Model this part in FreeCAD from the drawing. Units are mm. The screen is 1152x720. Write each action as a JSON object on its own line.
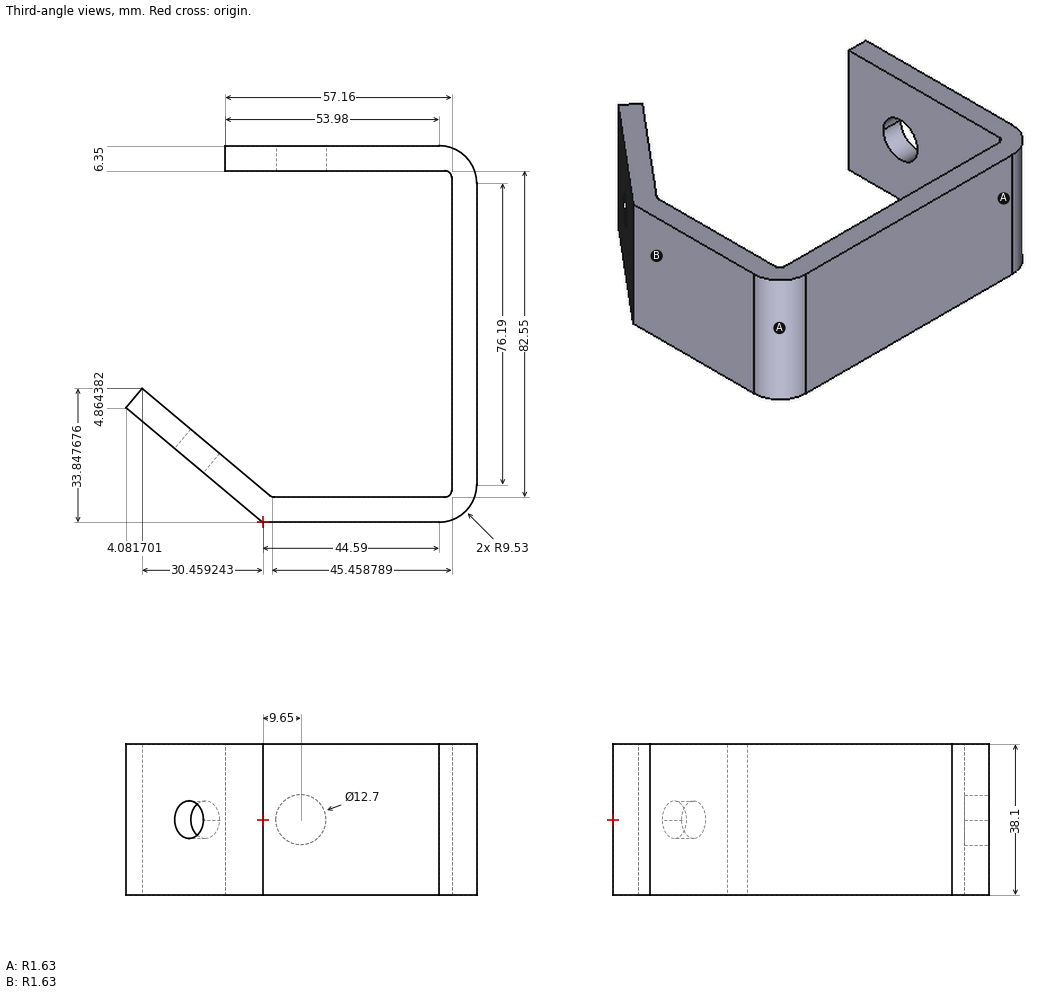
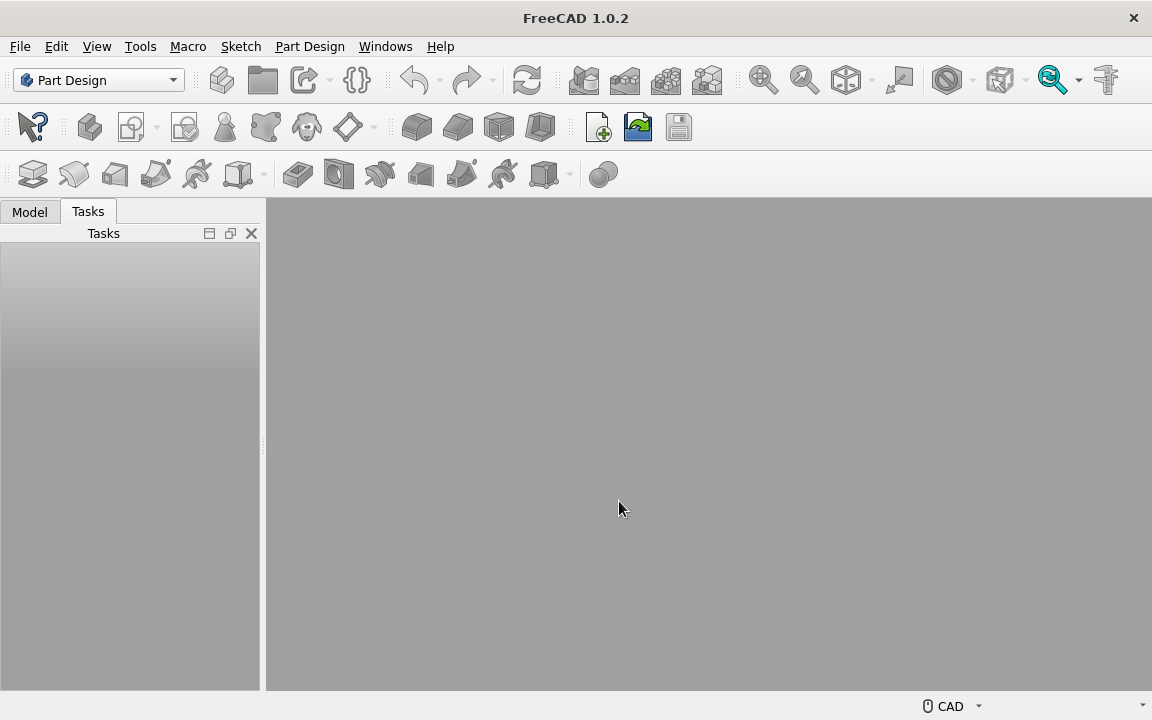
{"action": "key", "text": "ctrl+n"}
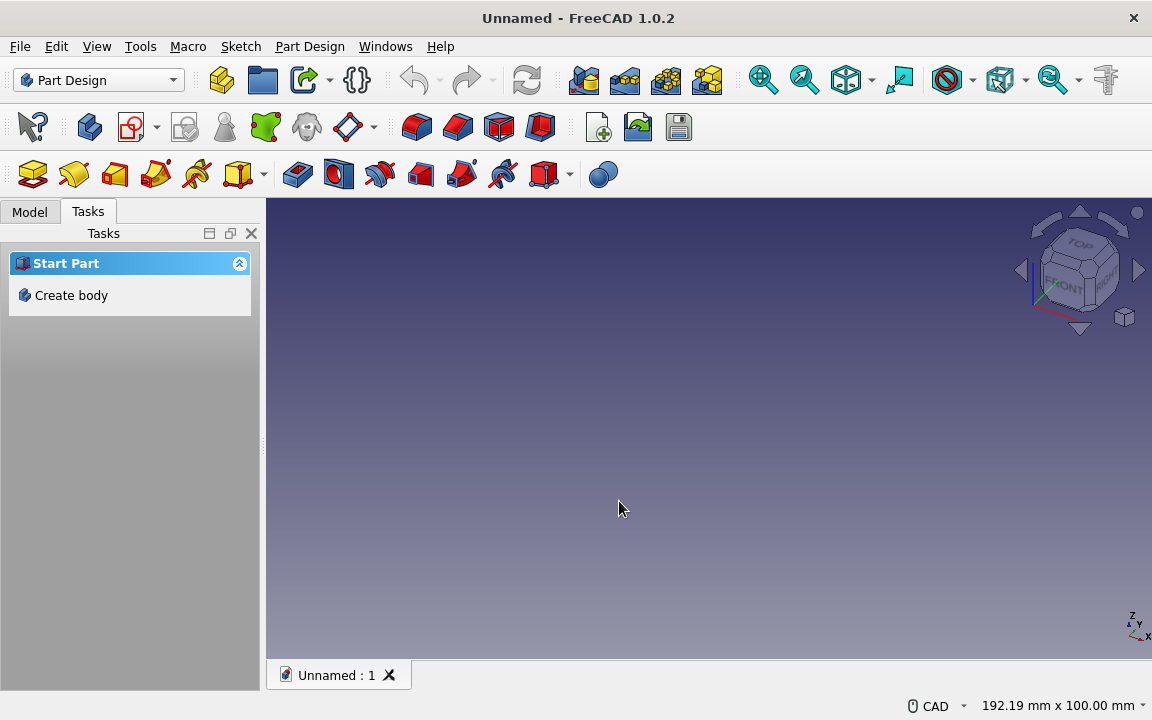
{"action": "left_click", "coordinate": [130, 128]}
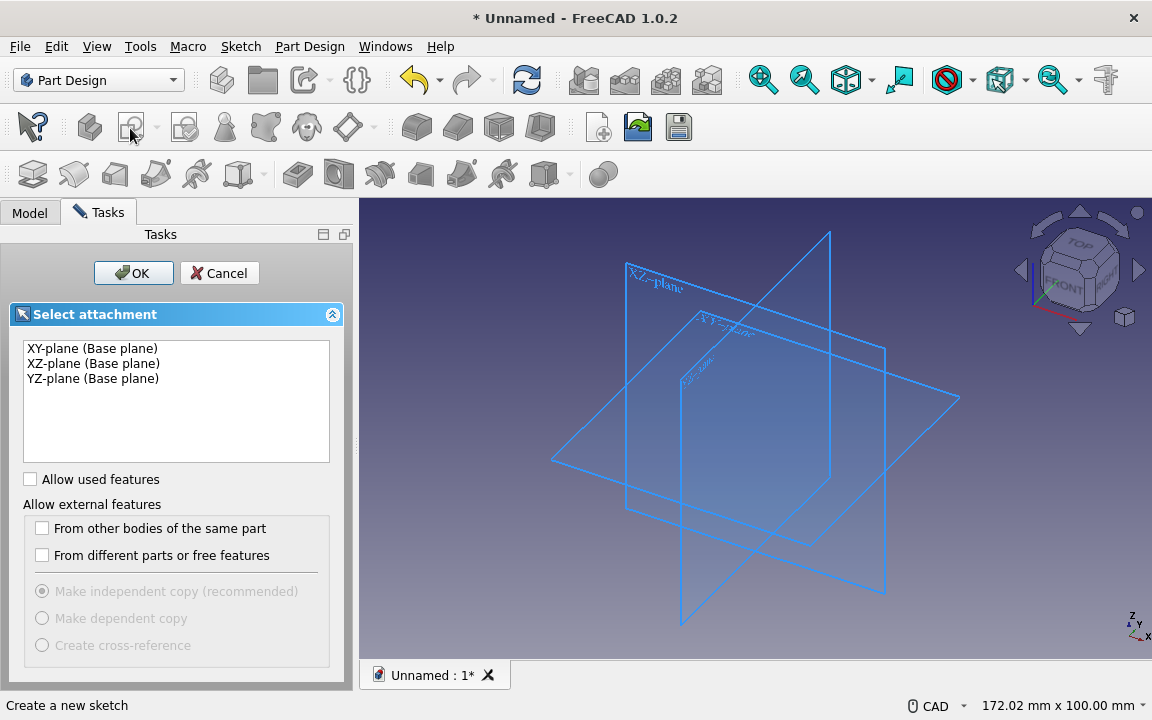
{"action": "left_click", "coordinate": [84, 348]}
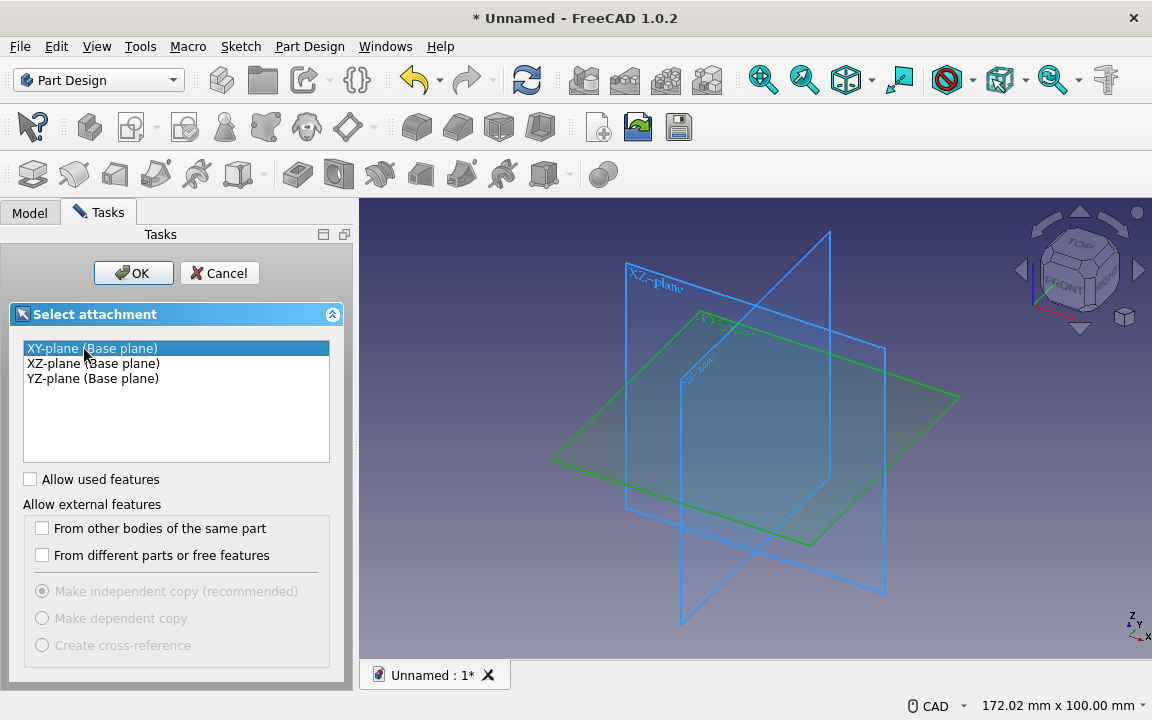
{"action": "left_click", "coordinate": [134, 273]}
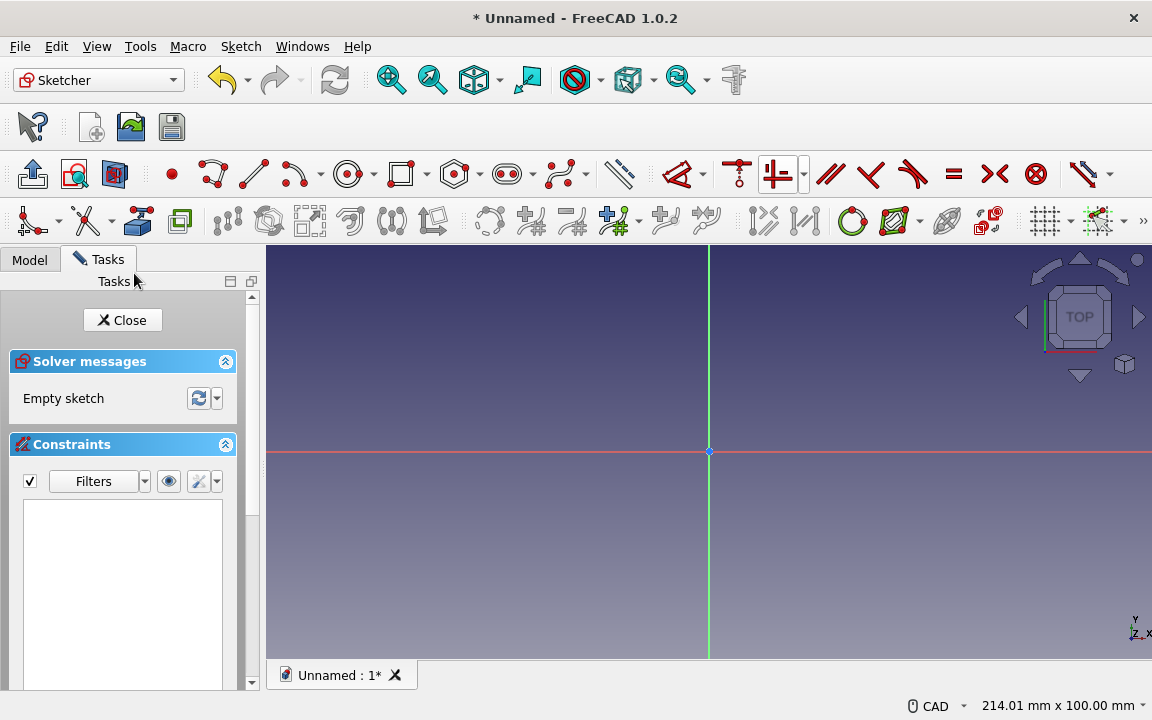
{"action": "scroll", "coordinate": [508, 631], "scroll_direction": "down", "scroll_amount": 3}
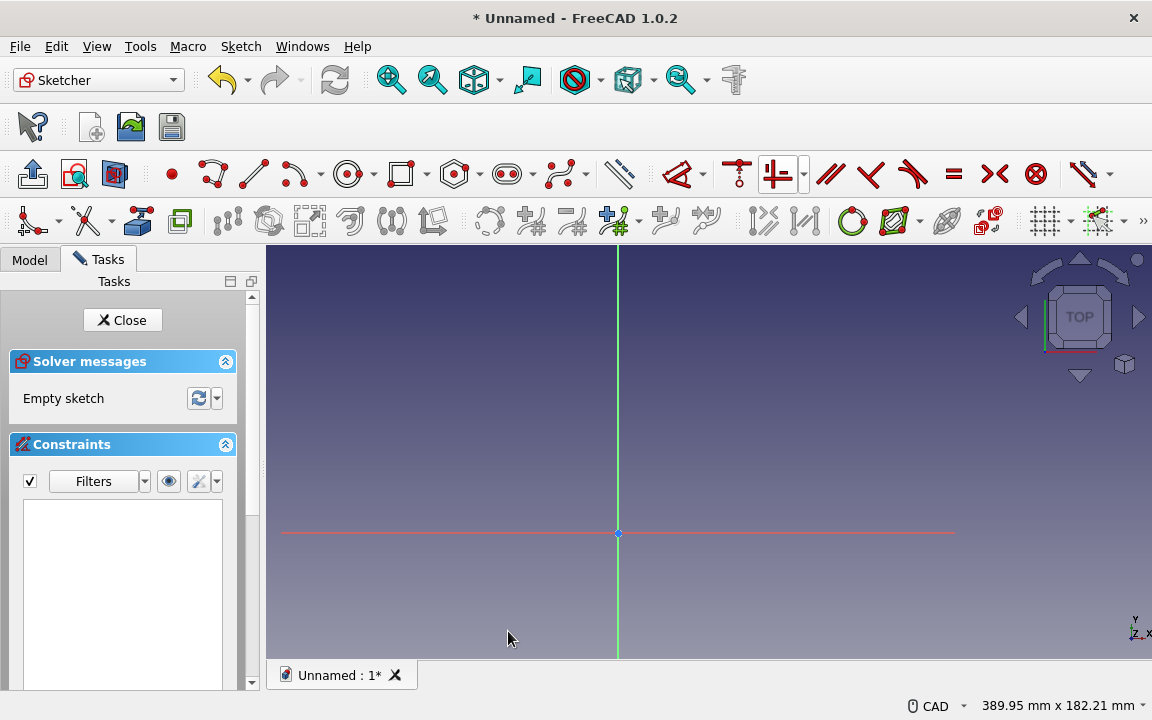
{"action": "key", "text": "g l"}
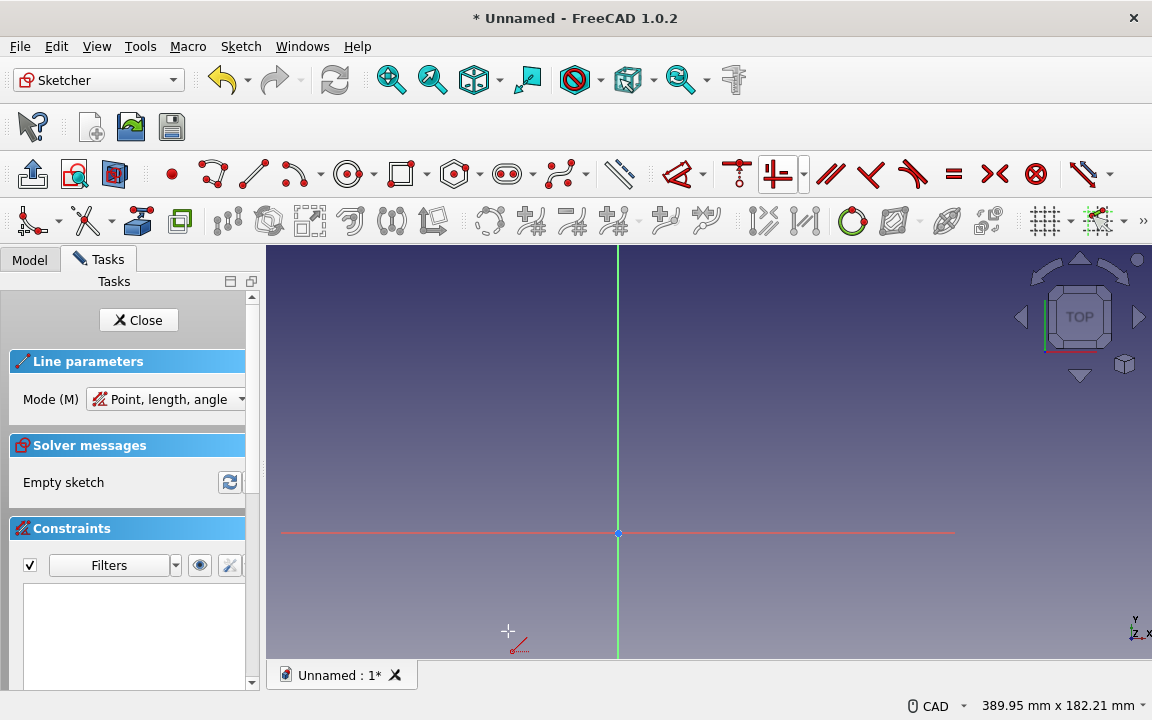
{"action": "left_click", "coordinate": [741, 512]}
{"action": "left_click", "coordinate": [741, 338]}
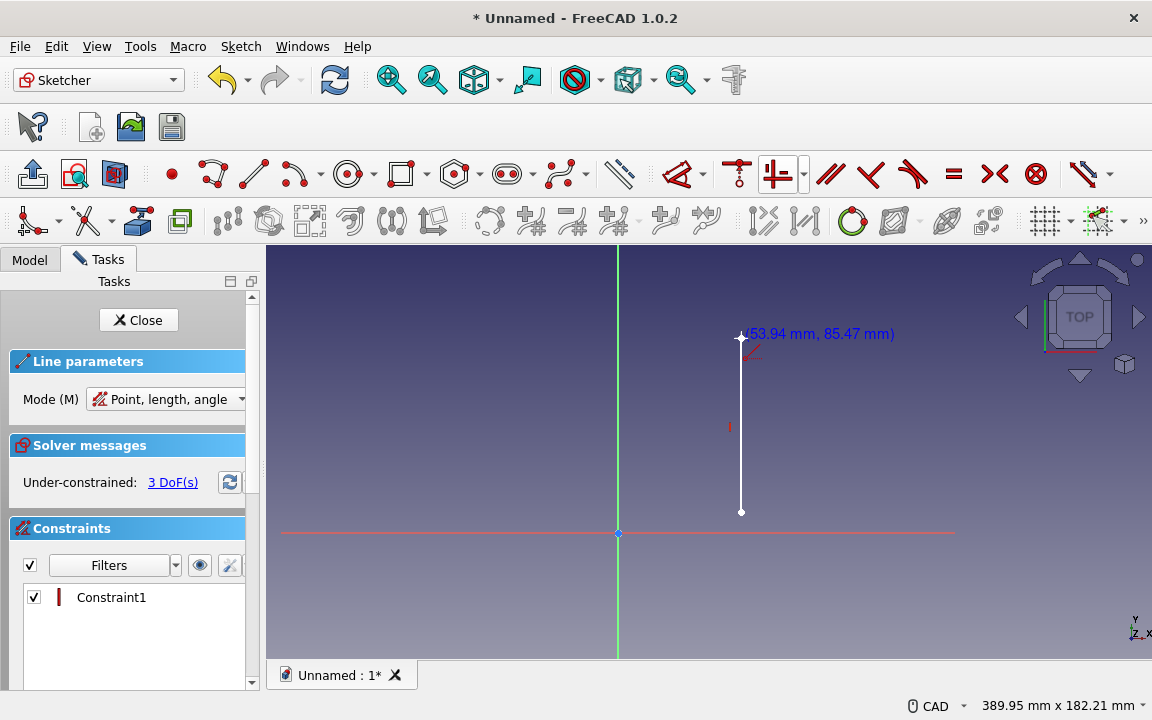
{"action": "key", "text": "g m"}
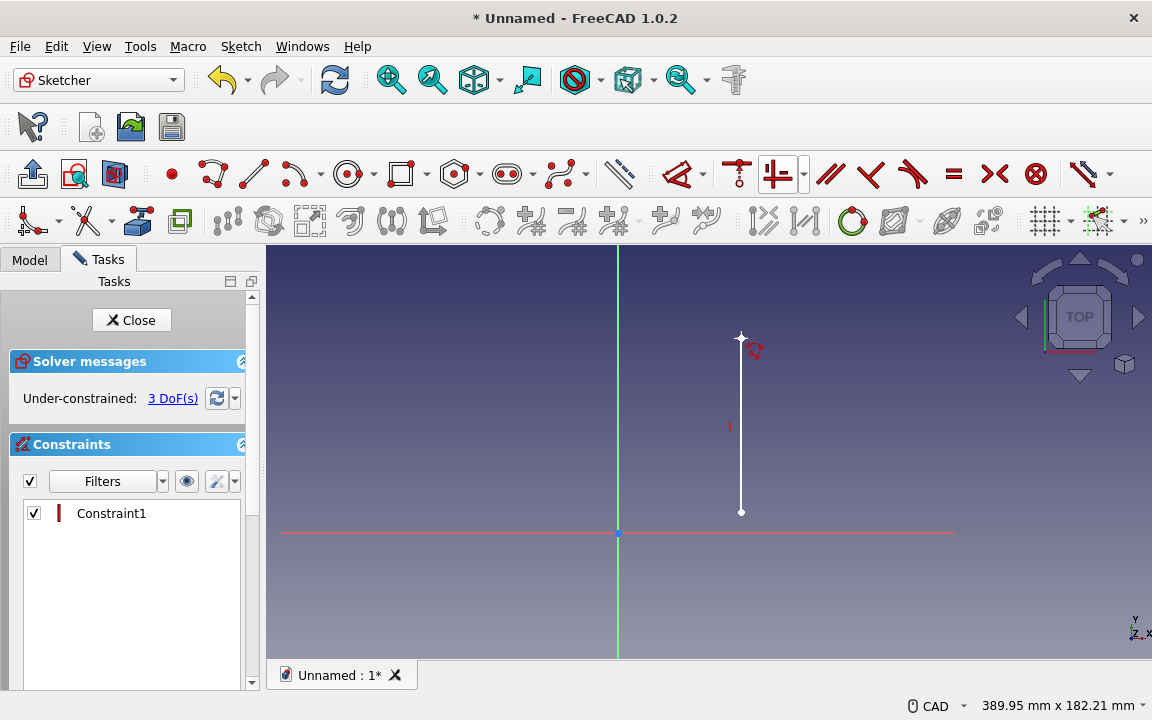
{"action": "left_click", "coordinate": [720, 317]}
{"action": "left_click", "coordinate": [597, 317]}
{"action": "left_click", "coordinate": [597, 331]}
{"action": "left_click", "coordinate": [727, 331]}
{"action": "left_click", "coordinate": [727, 519]}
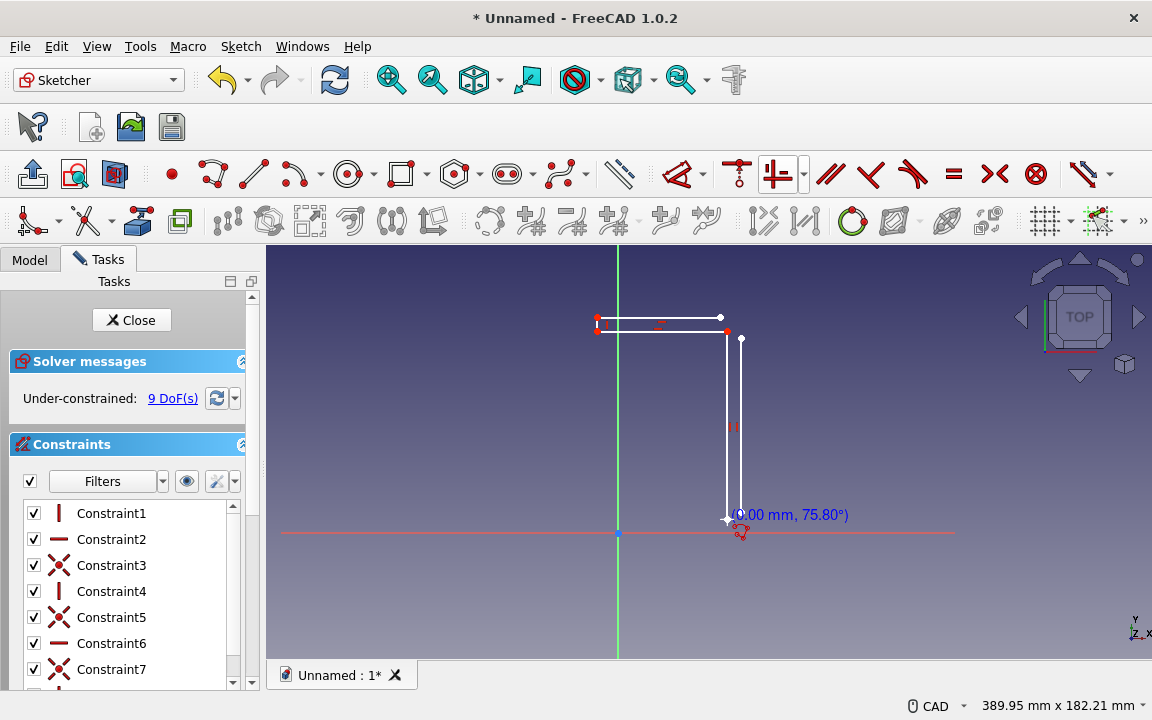
{"action": "scroll", "coordinate": [624, 519], "scroll_direction": "up", "scroll_amount": 6}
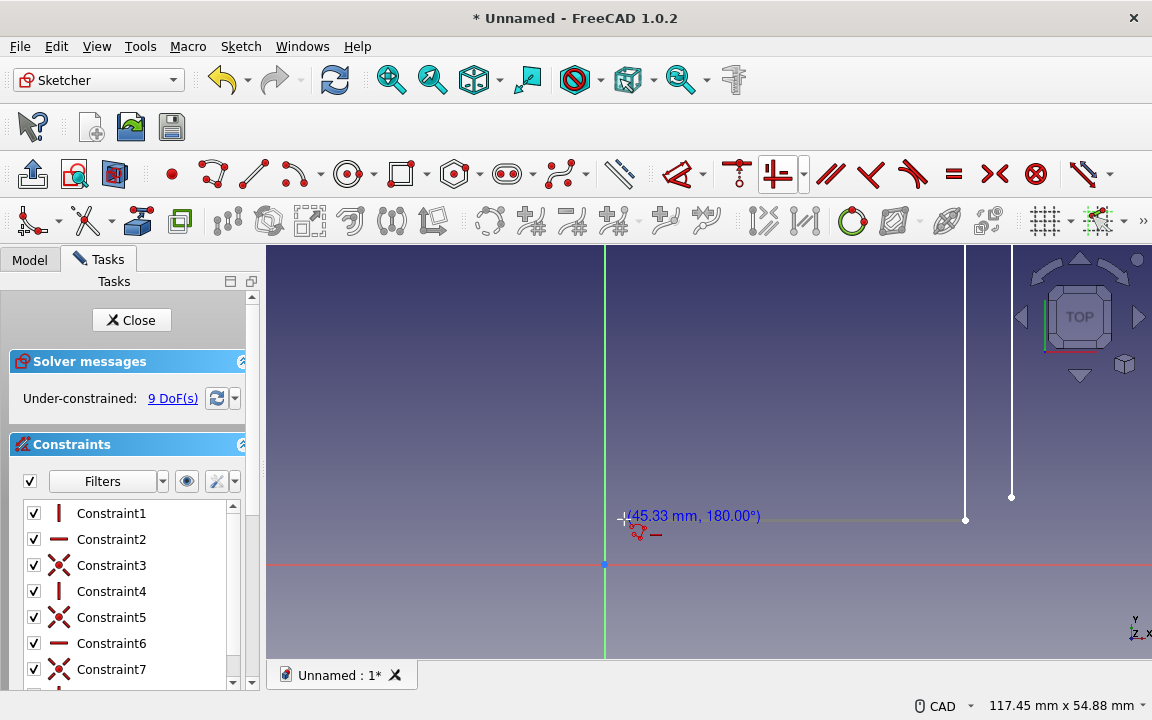
{"action": "left_click", "coordinate": [622, 517]}
{"action": "left_click", "coordinate": [375, 309]}
{"action": "left_click", "coordinate": [344, 346]}
{"action": "left_click", "coordinate": [605, 565]}
{"action": "left_click", "coordinate": [941, 556]}
{"action": "right_click", "coordinate": [941, 556]}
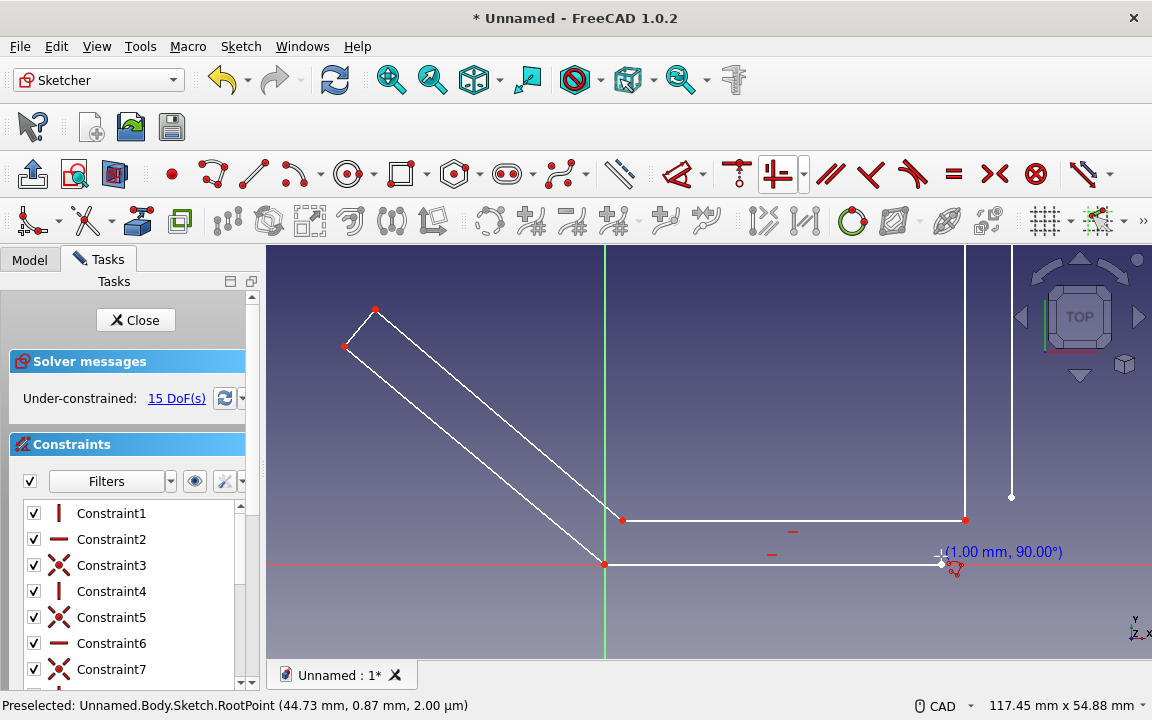
{"action": "key", "text": "g 3 a"}